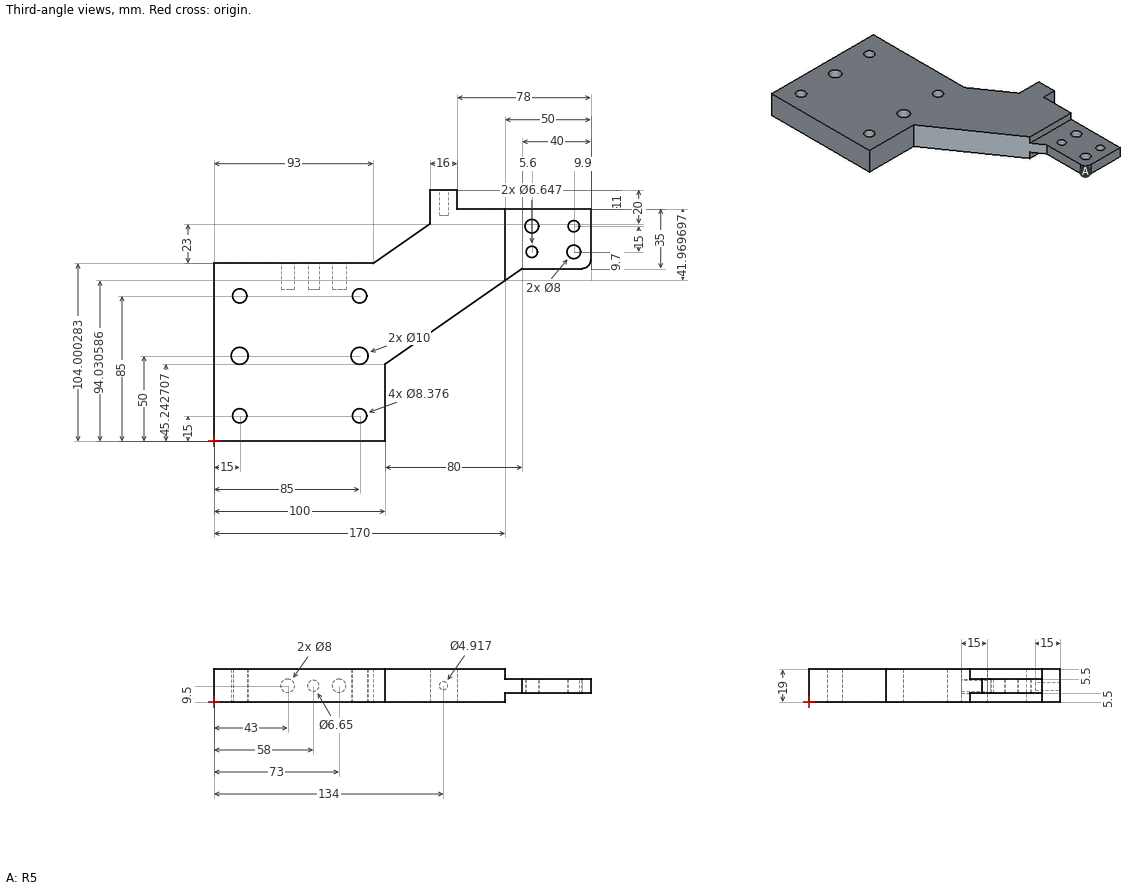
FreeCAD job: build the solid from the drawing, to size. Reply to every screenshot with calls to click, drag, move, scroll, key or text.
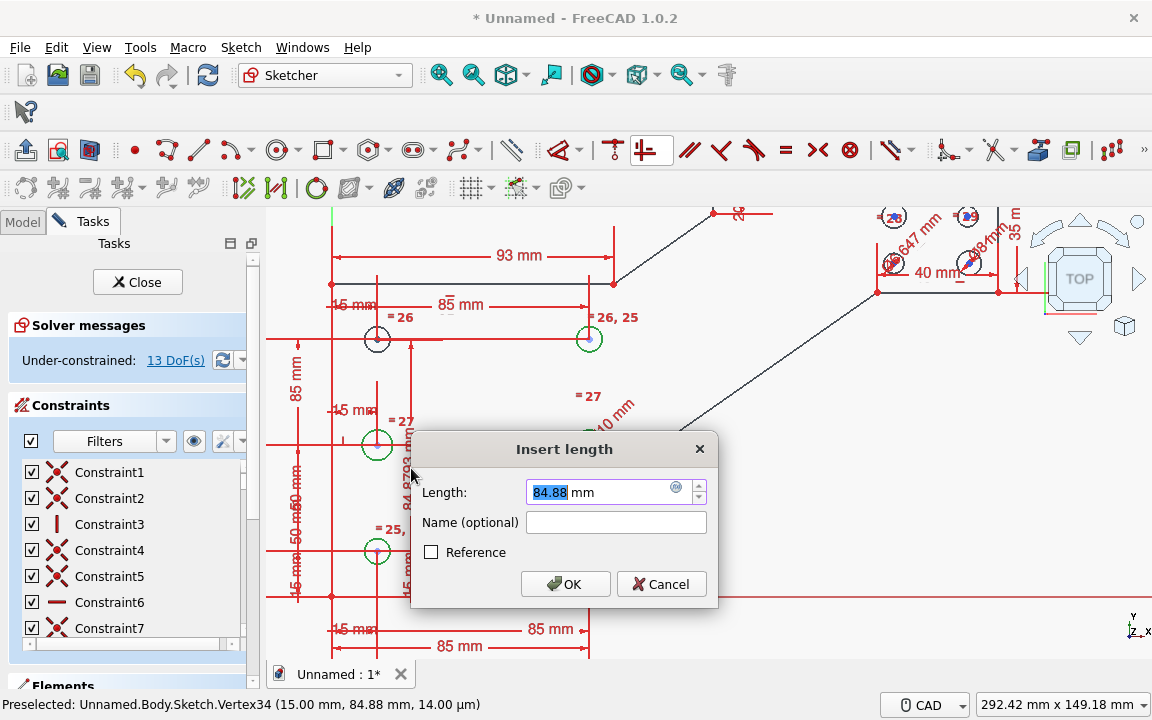
text(85)
key(Return)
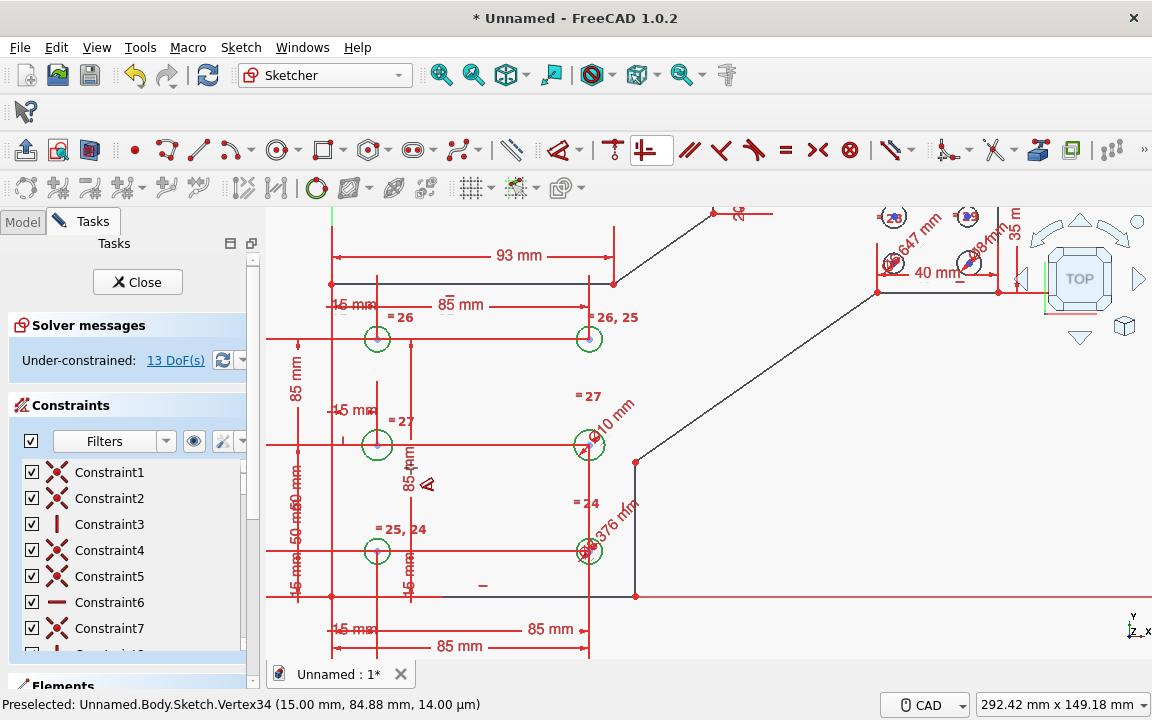
click(423, 597)
click(484, 563)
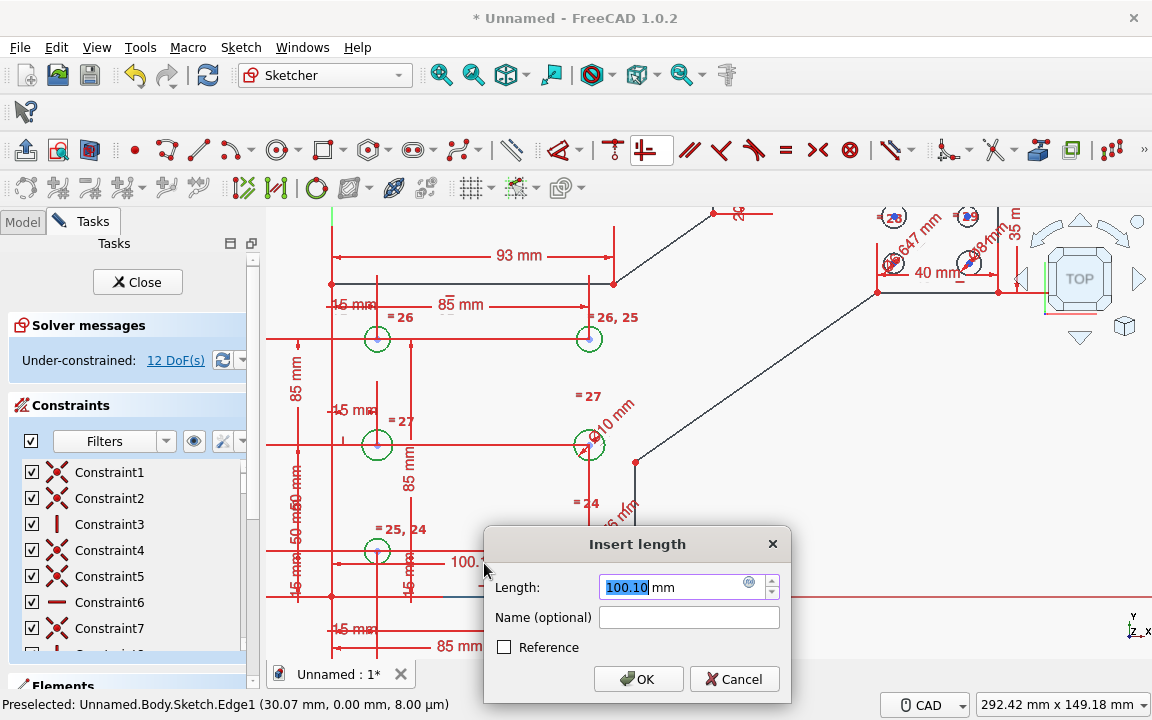
text(100)
key(Return)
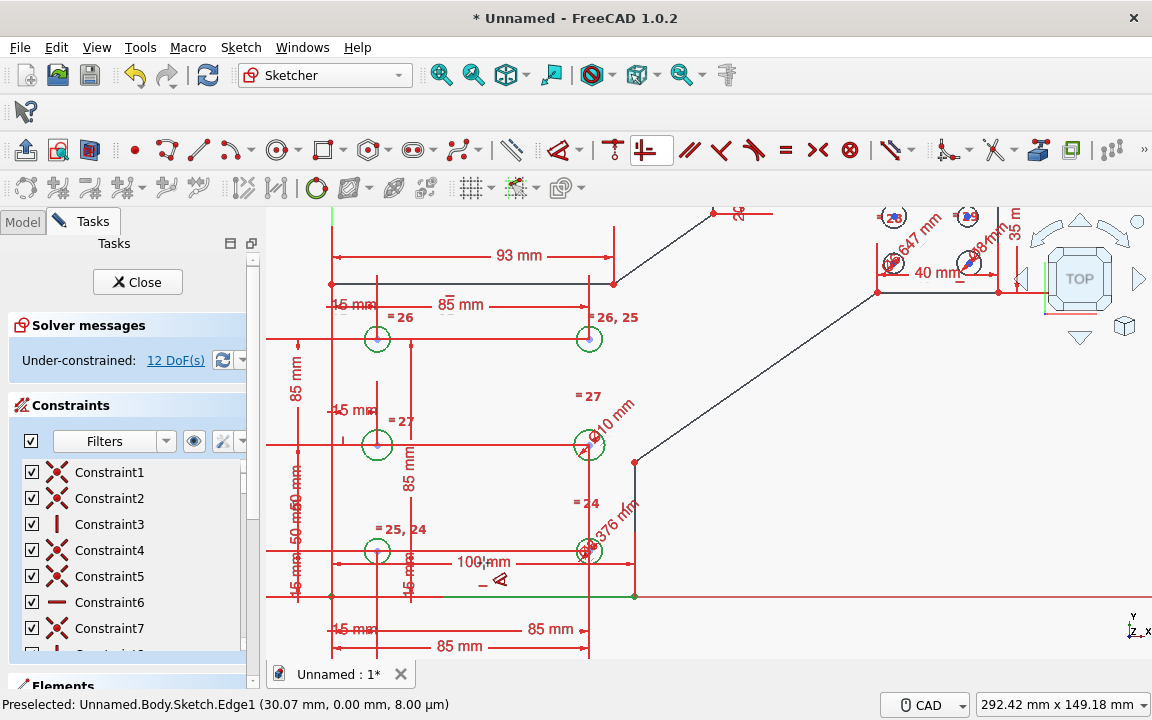
click(708, 411)
click(756, 496)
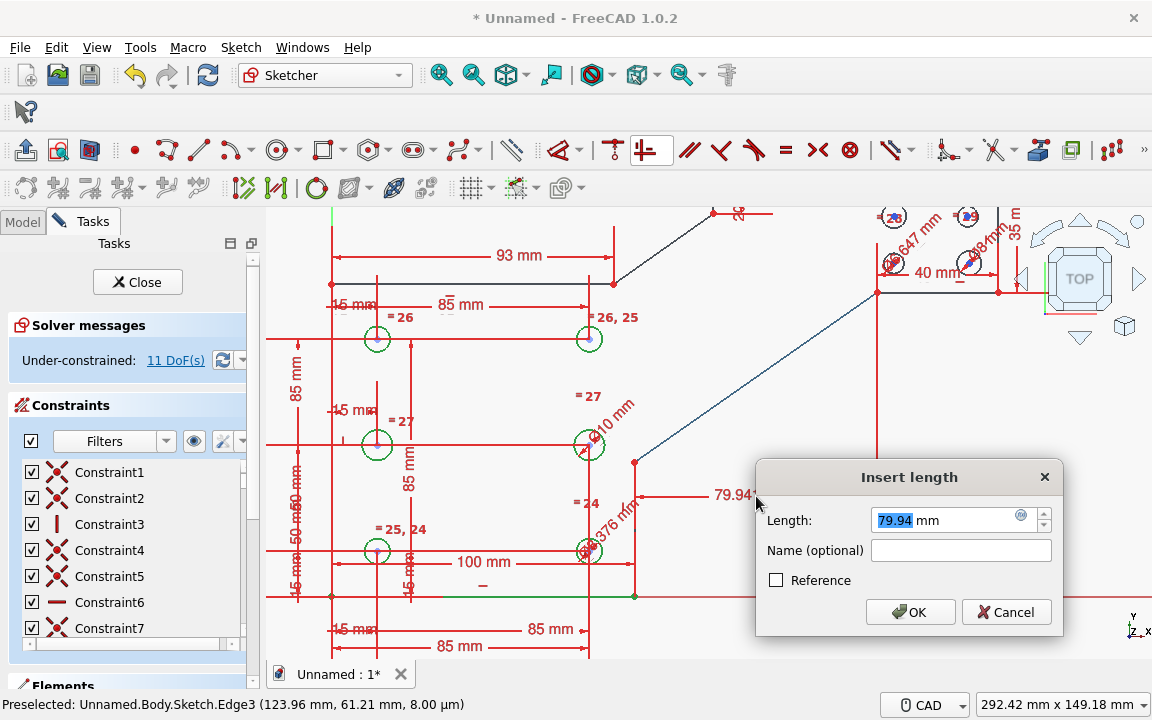
text(80)
key(Return)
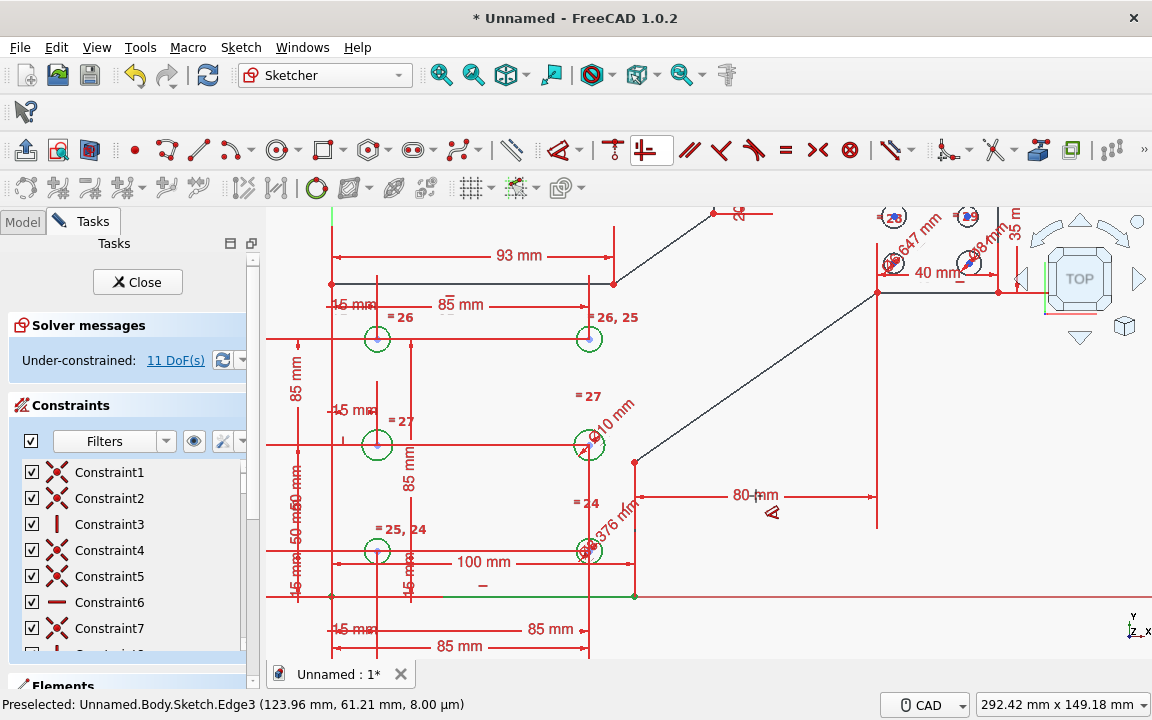
click(644, 263)
click(748, 260)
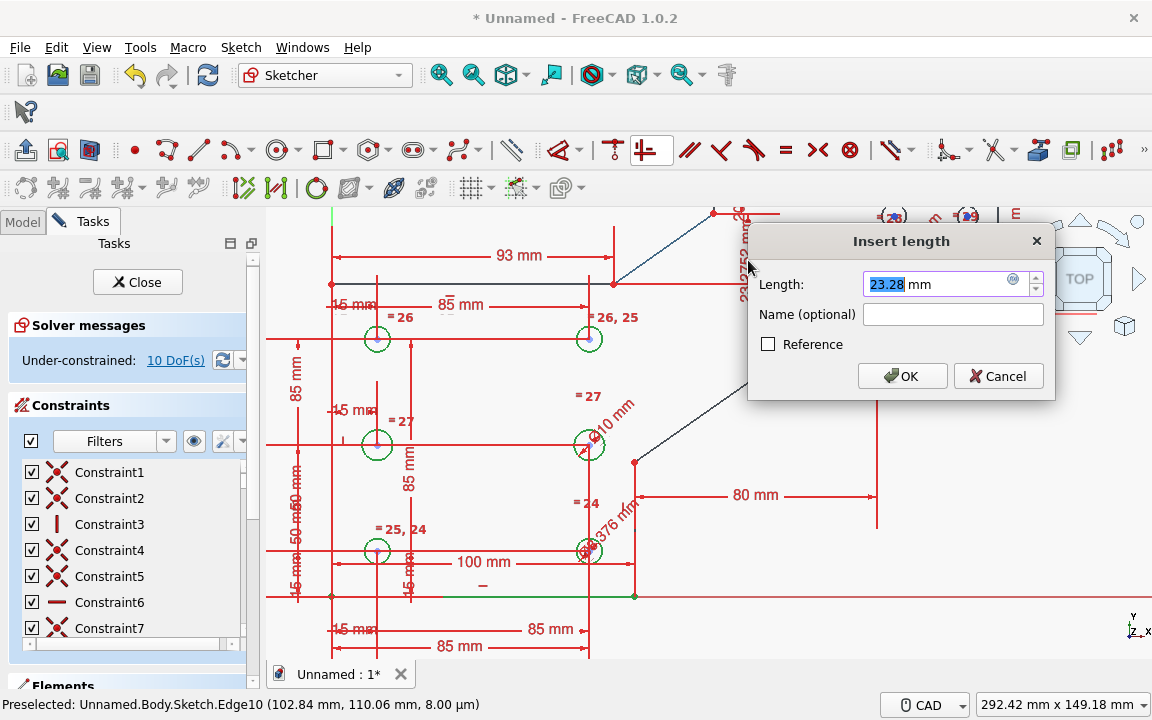
text(23)
key(Return)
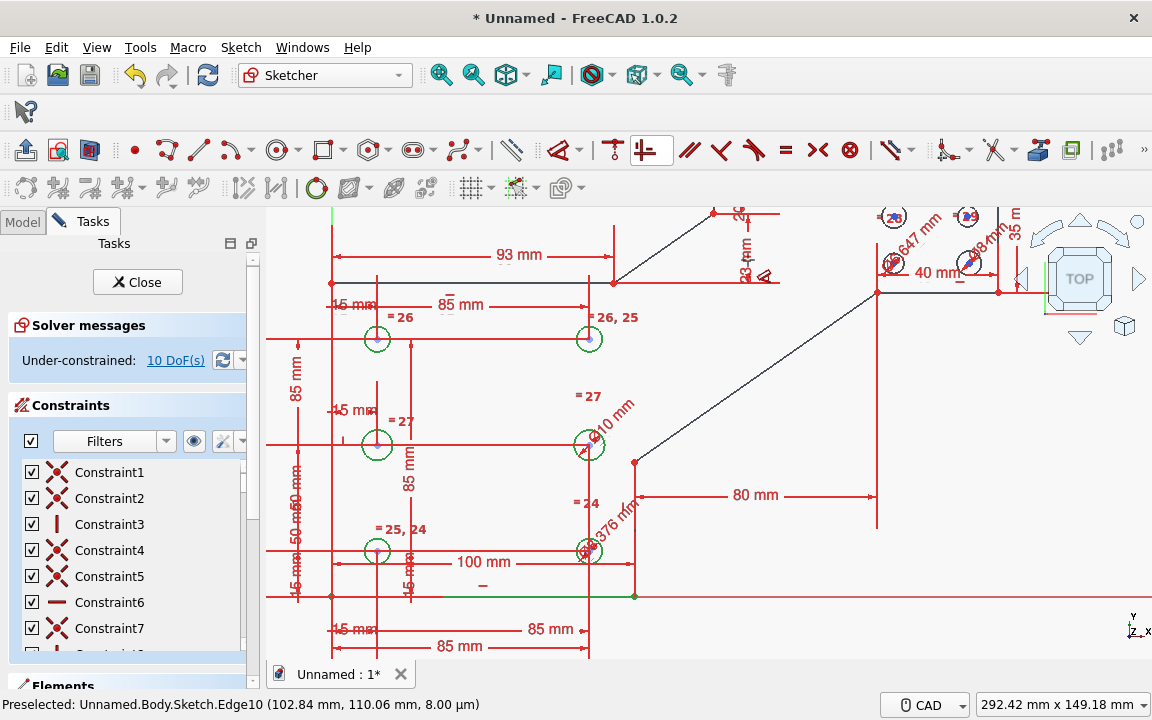
click(969, 263)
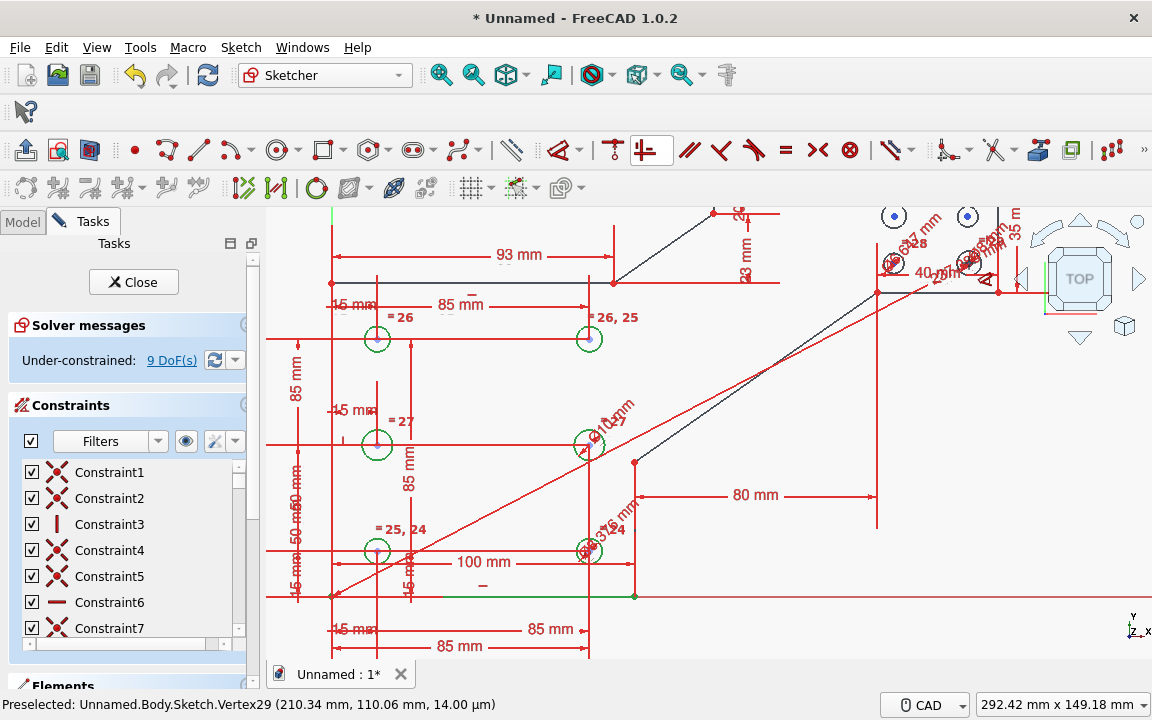
scroll(590, 553, down, 2)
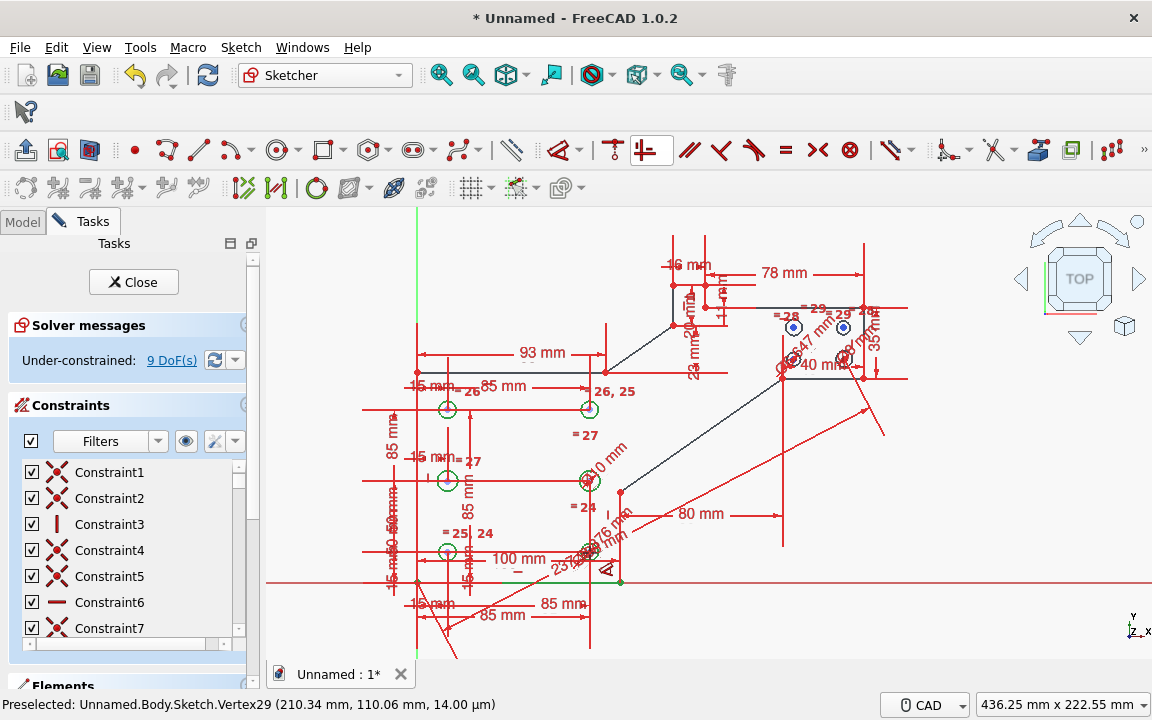
scroll(843, 328, up, 2)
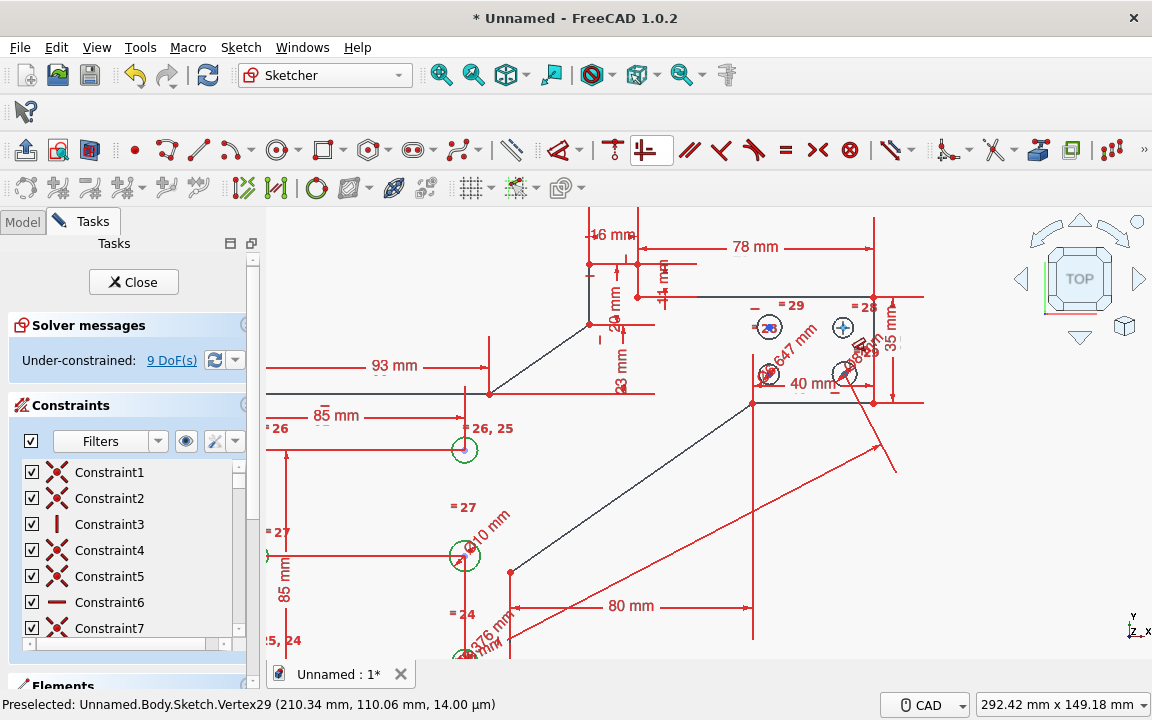
click(843, 328)
click(951, 351)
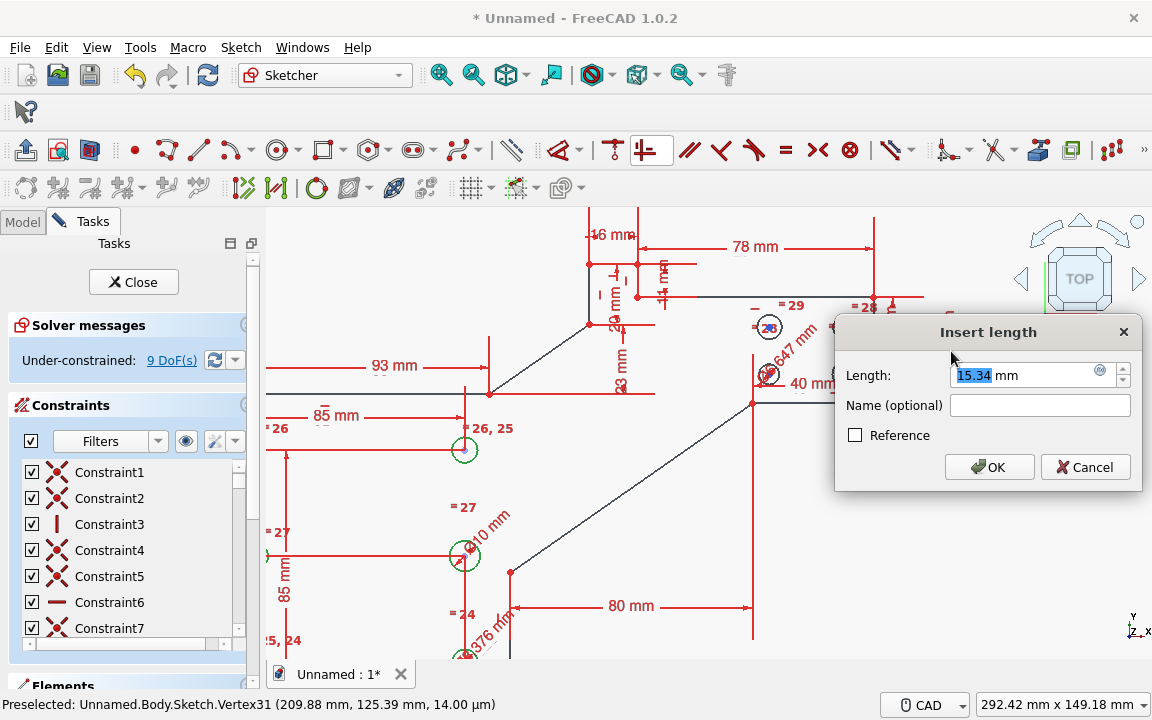
text(15)
key(Return)